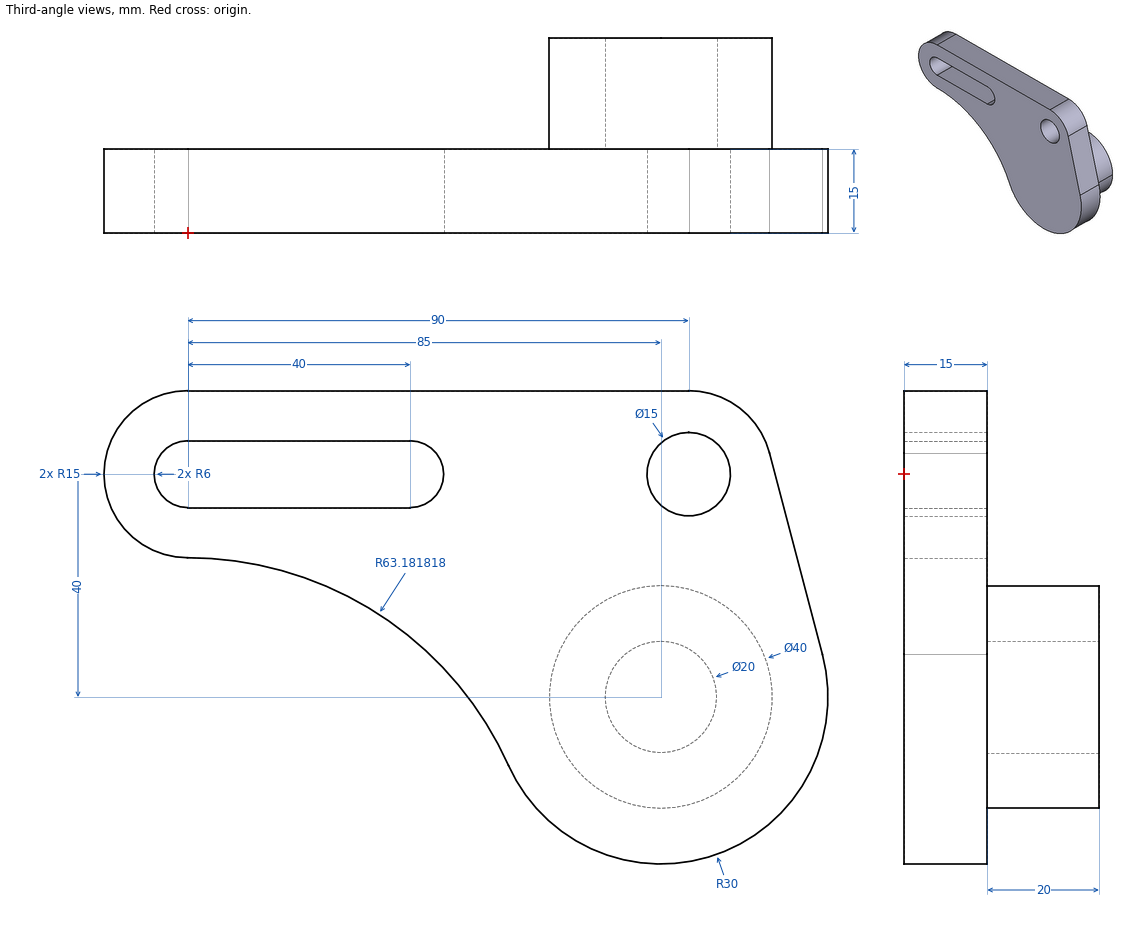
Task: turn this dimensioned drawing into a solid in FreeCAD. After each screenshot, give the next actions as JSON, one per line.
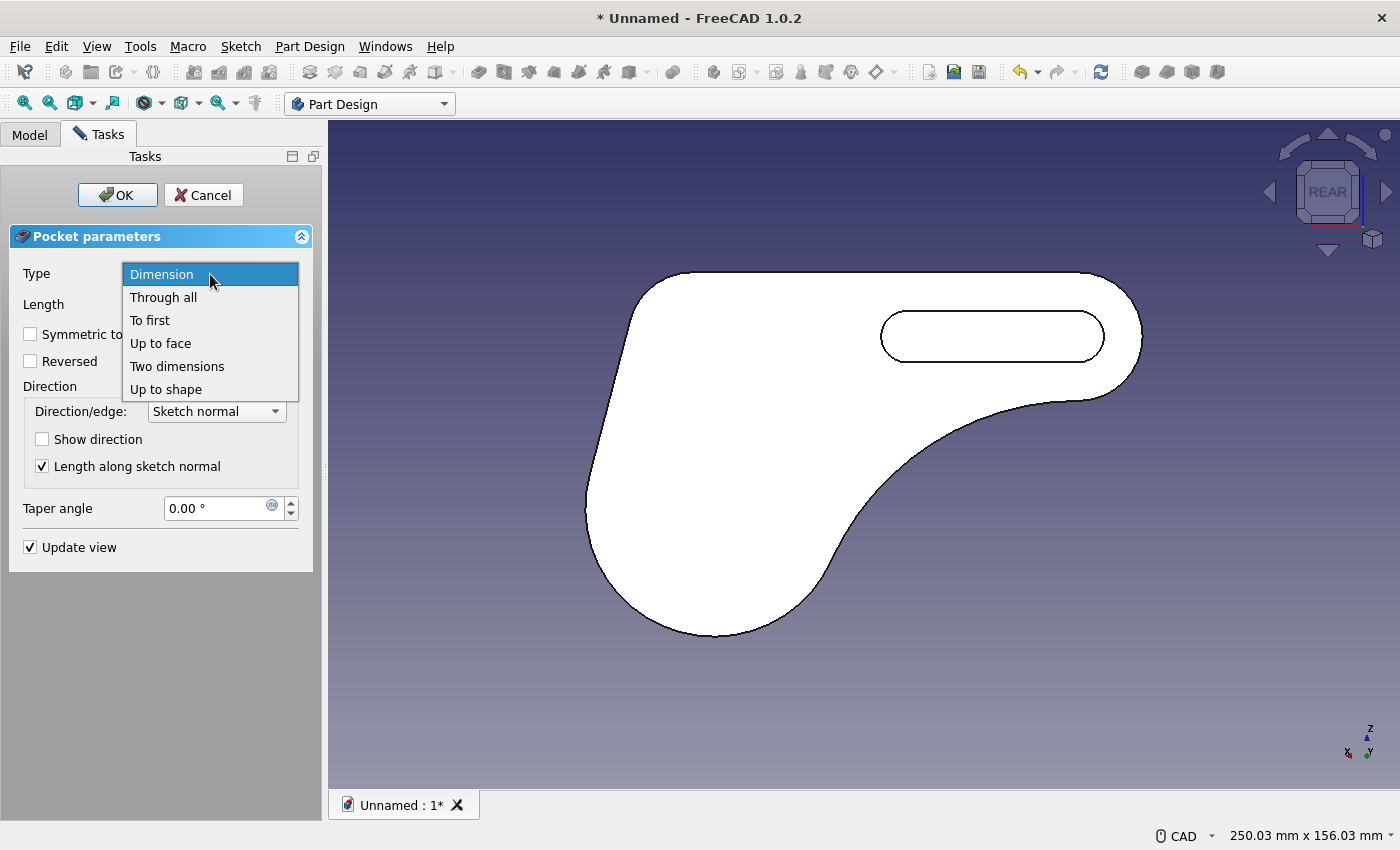
{"action": "left_click", "coordinate": [208, 298]}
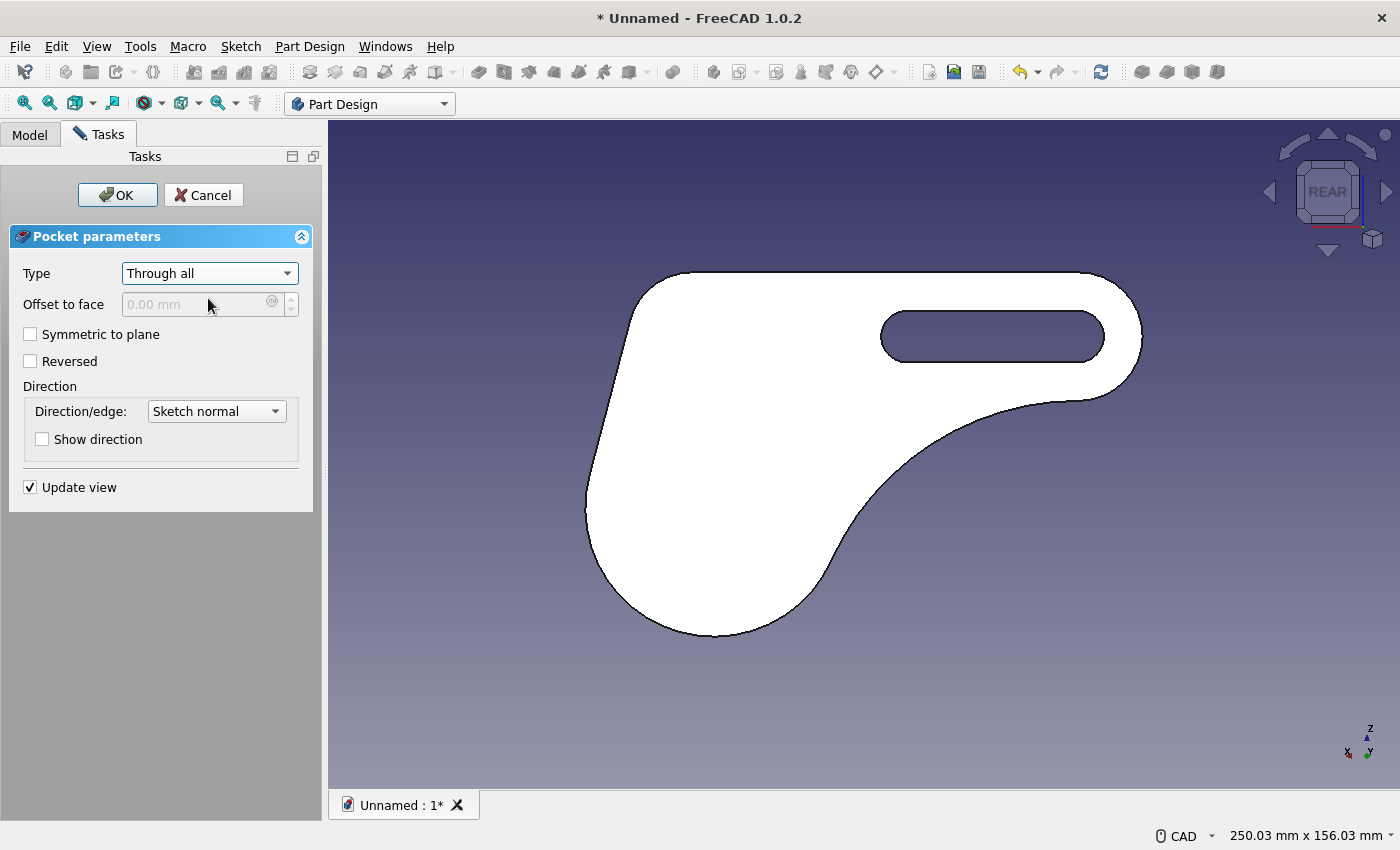
{"action": "left_click", "coordinate": [118, 195]}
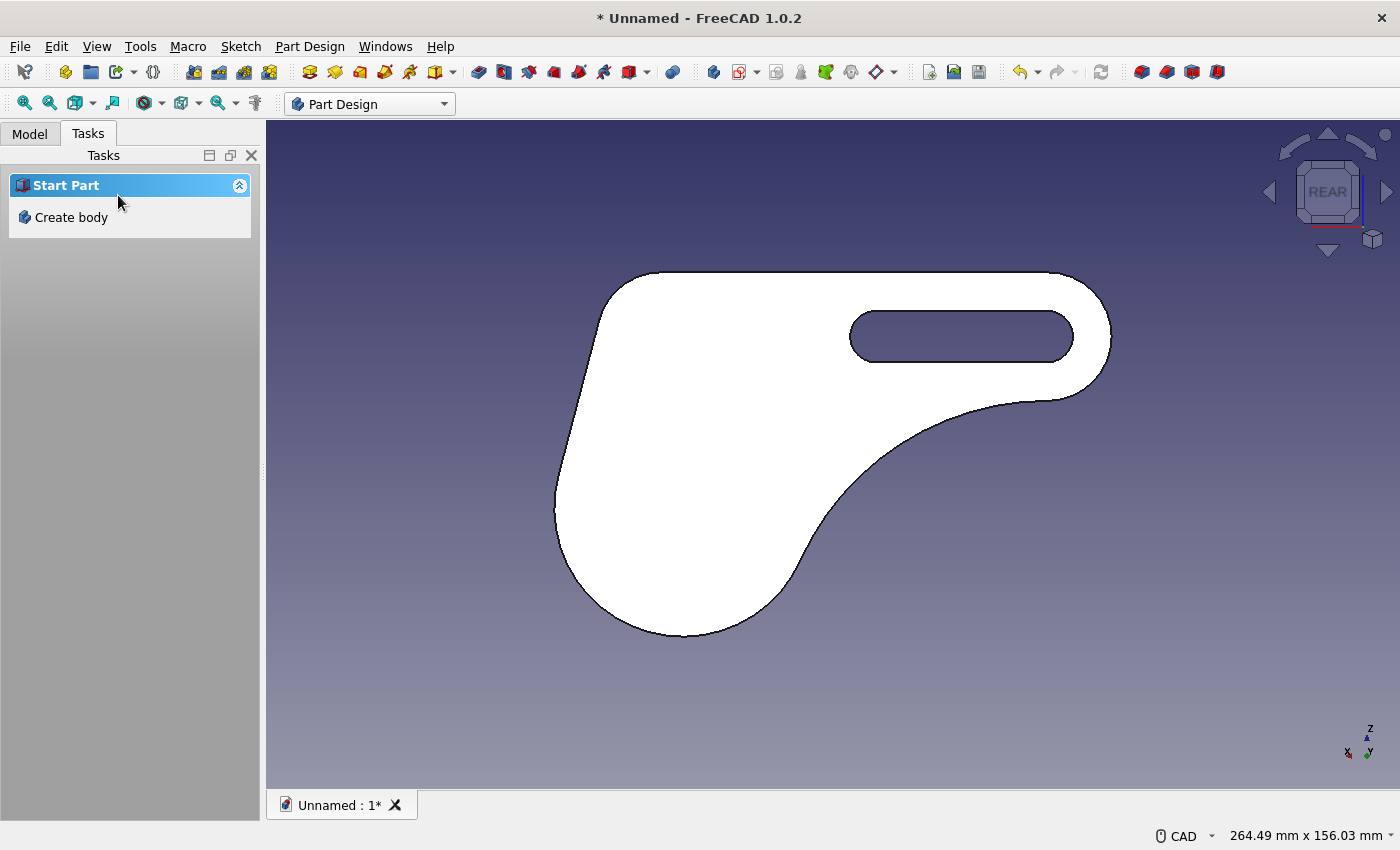
{"action": "left_click", "coordinate": [674, 506]}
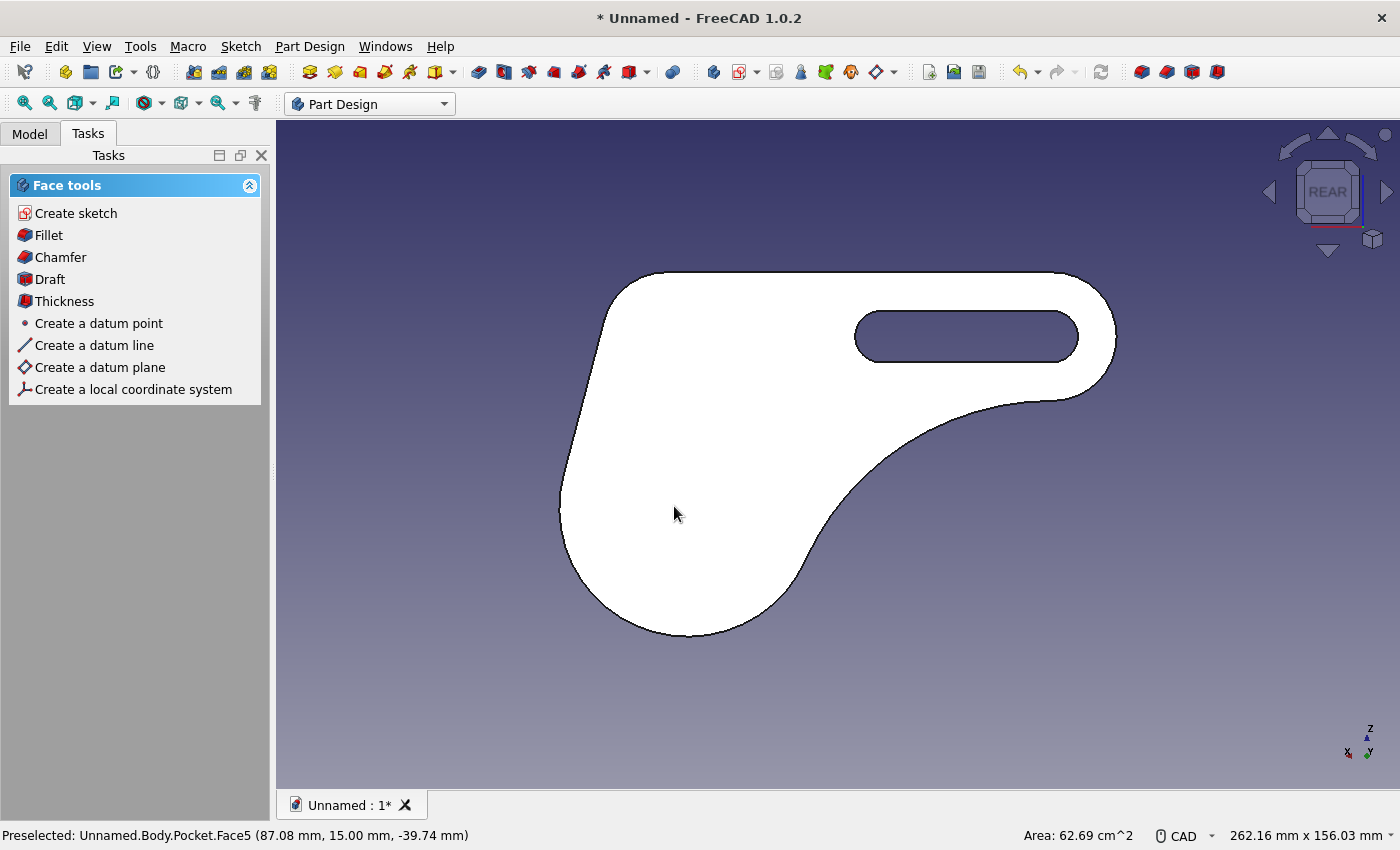
{"action": "left_click", "coordinate": [738, 72]}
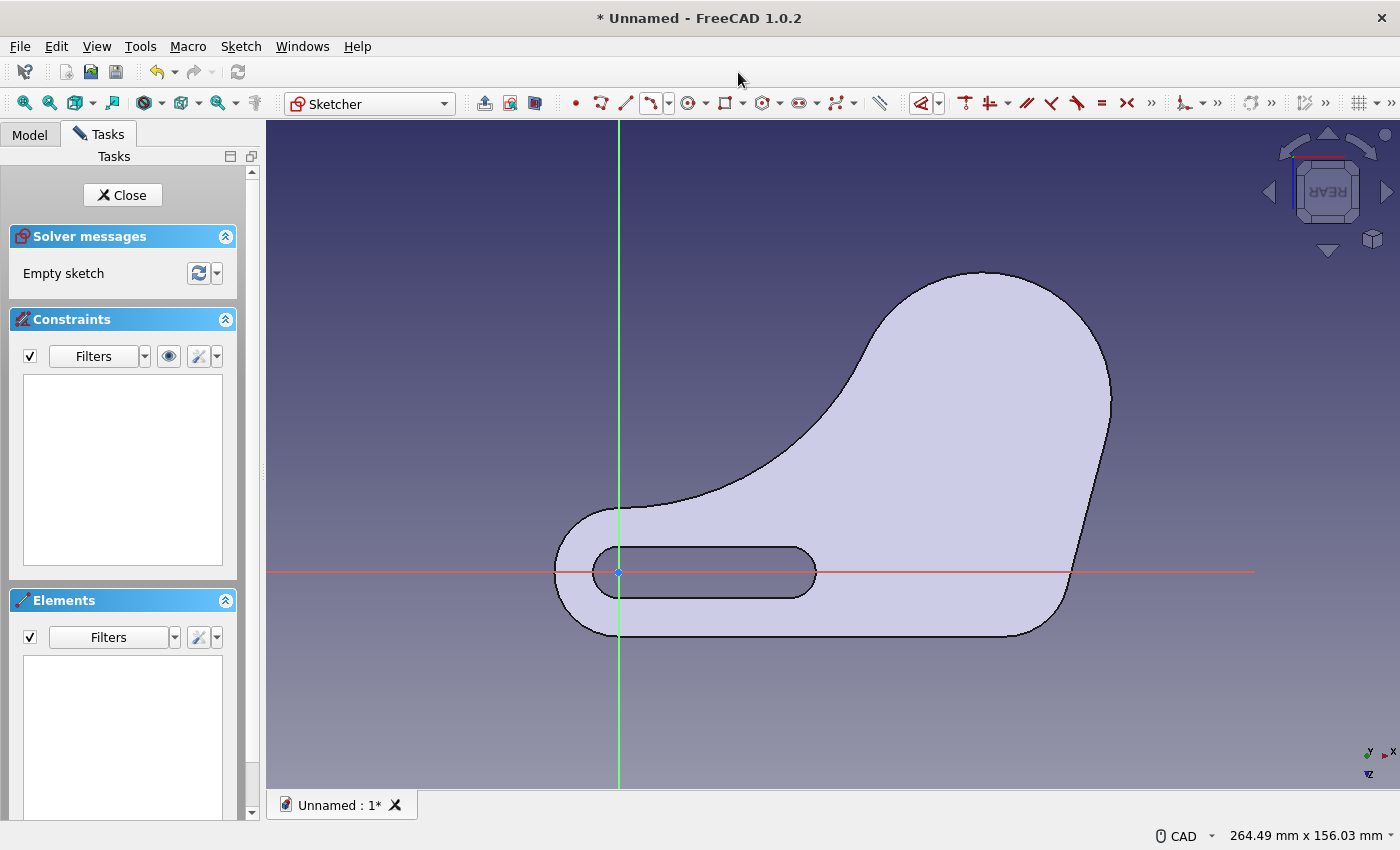
{"action": "scroll", "coordinate": [1042, 591], "scroll_direction": "up", "scroll_amount": 10}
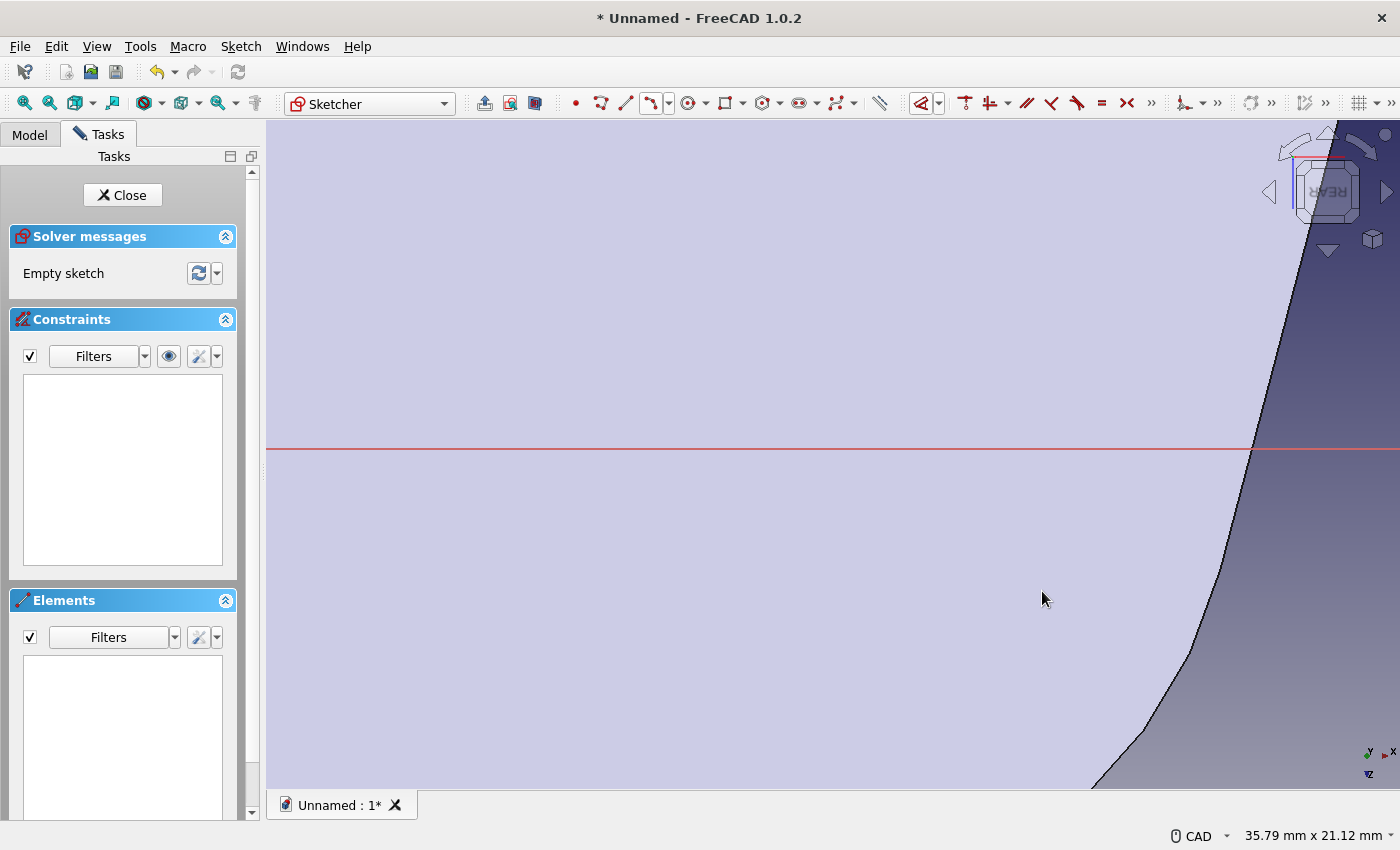
{"action": "left_click", "coordinate": [688, 104]}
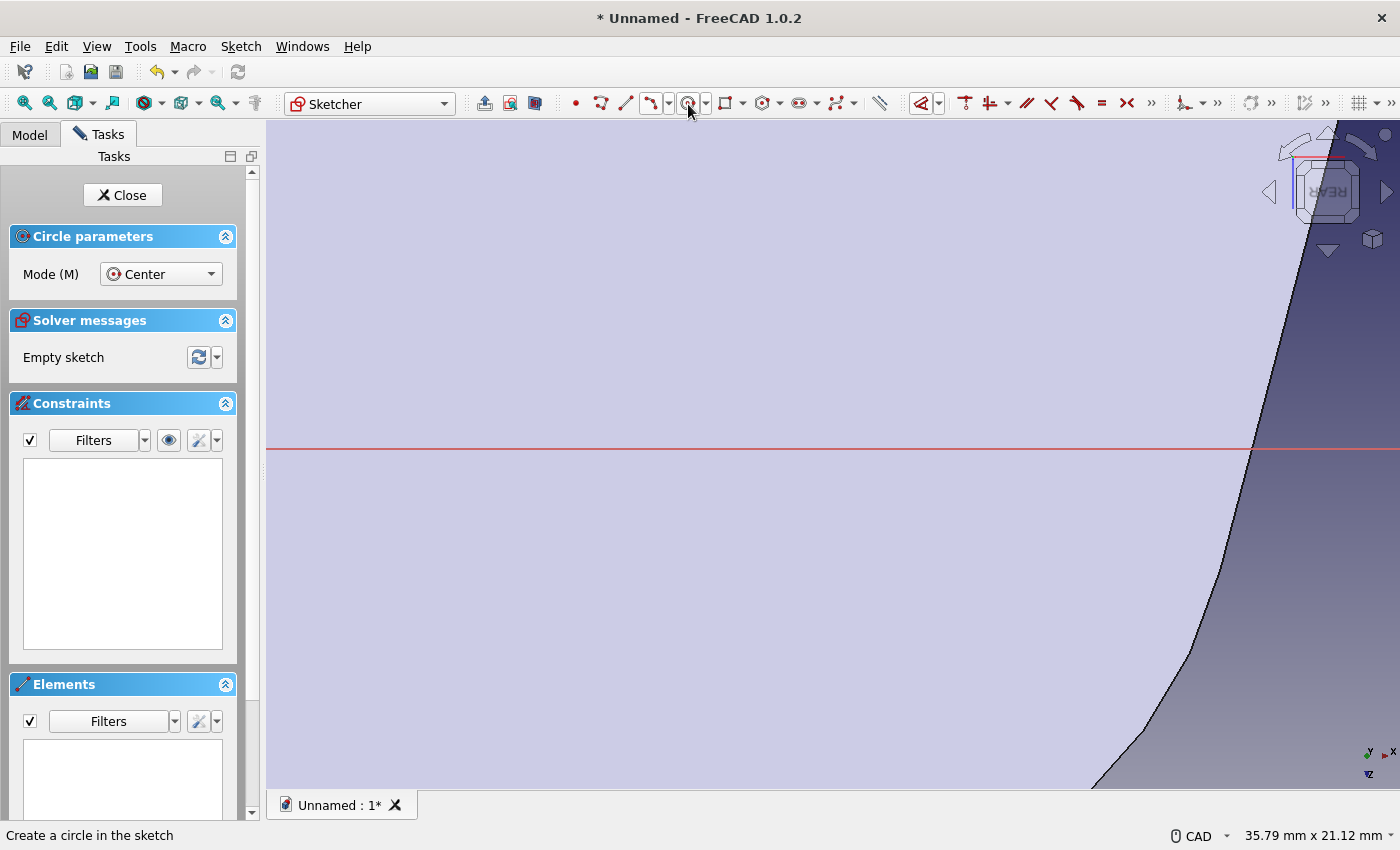
{"action": "left_click", "coordinate": [761, 449]}
{"action": "left_click", "coordinate": [929, 281]}
{"action": "key", "text": "Escape"}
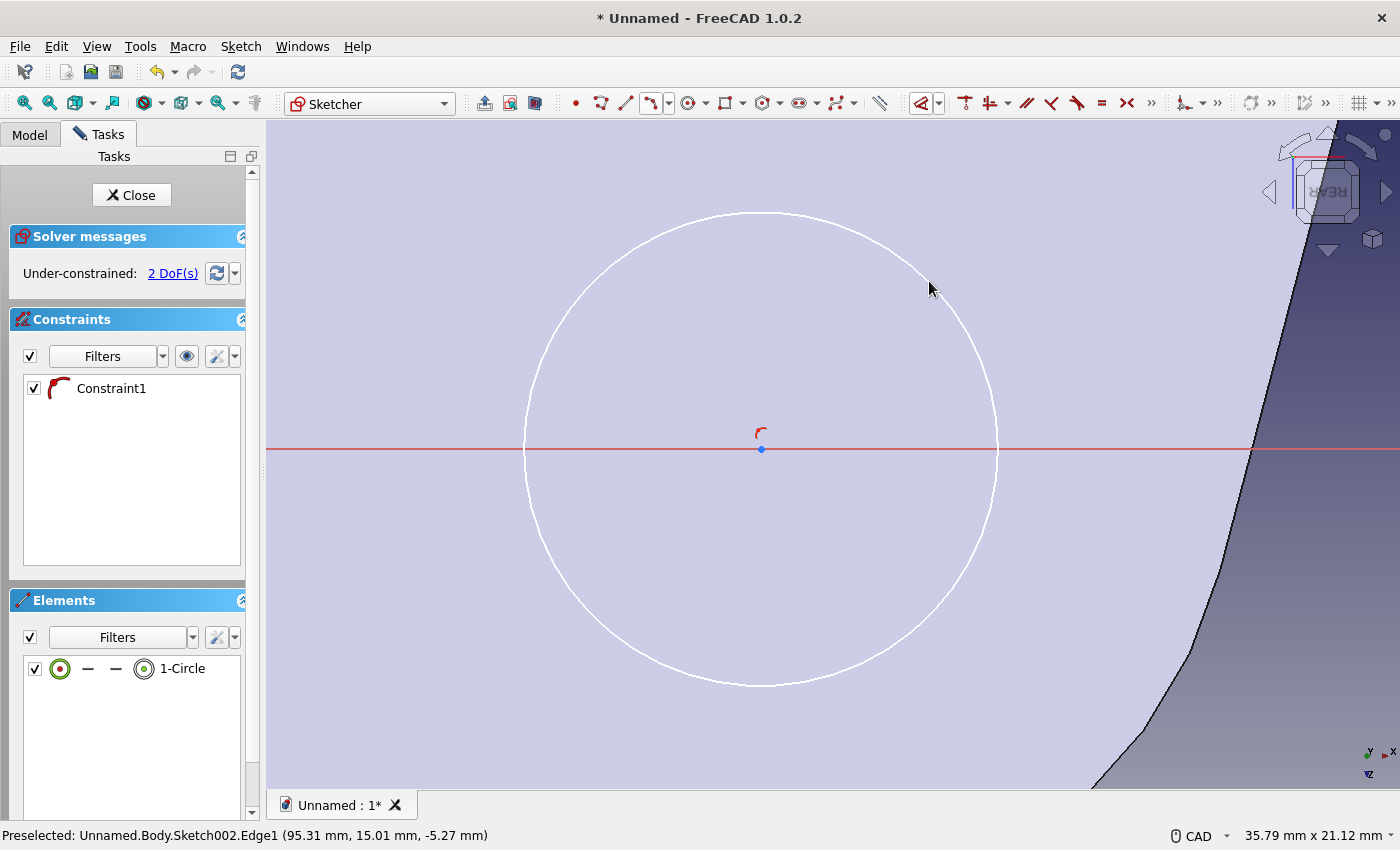
{"action": "left_click", "coordinate": [928, 281]}